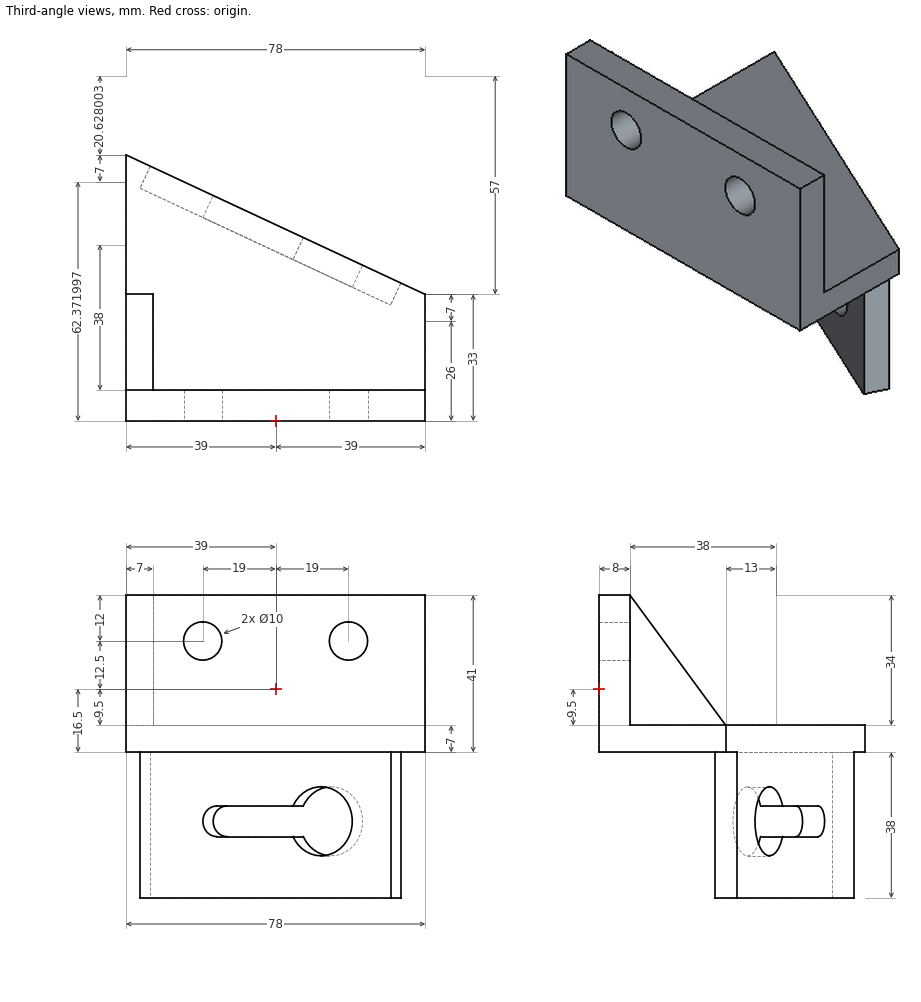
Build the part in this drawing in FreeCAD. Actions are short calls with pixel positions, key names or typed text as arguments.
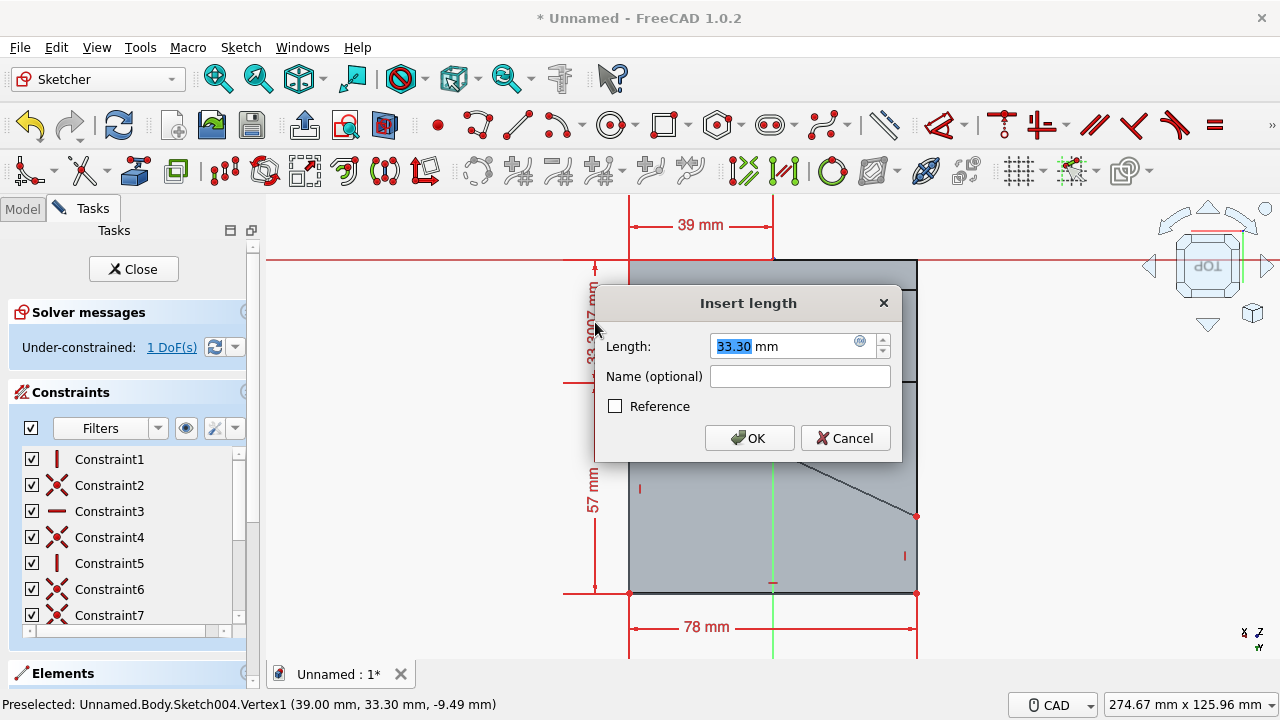
text(33)
key(Return)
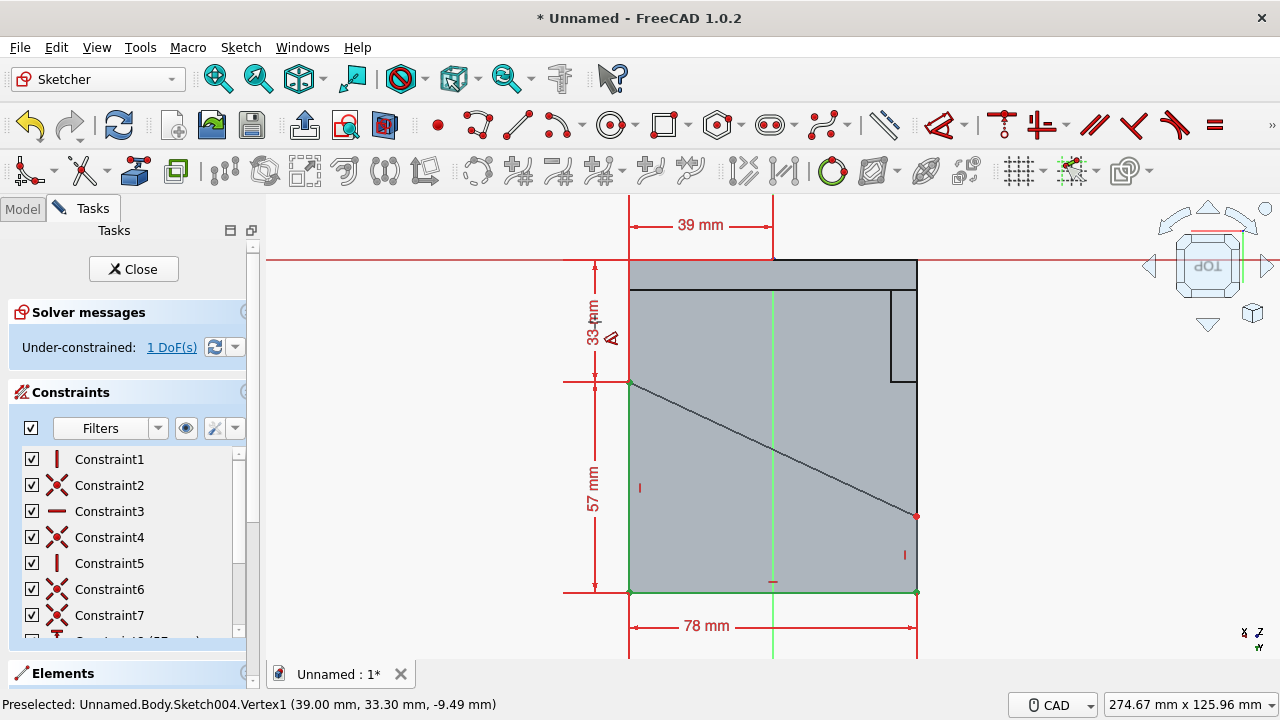
click(917, 570)
click(951, 555)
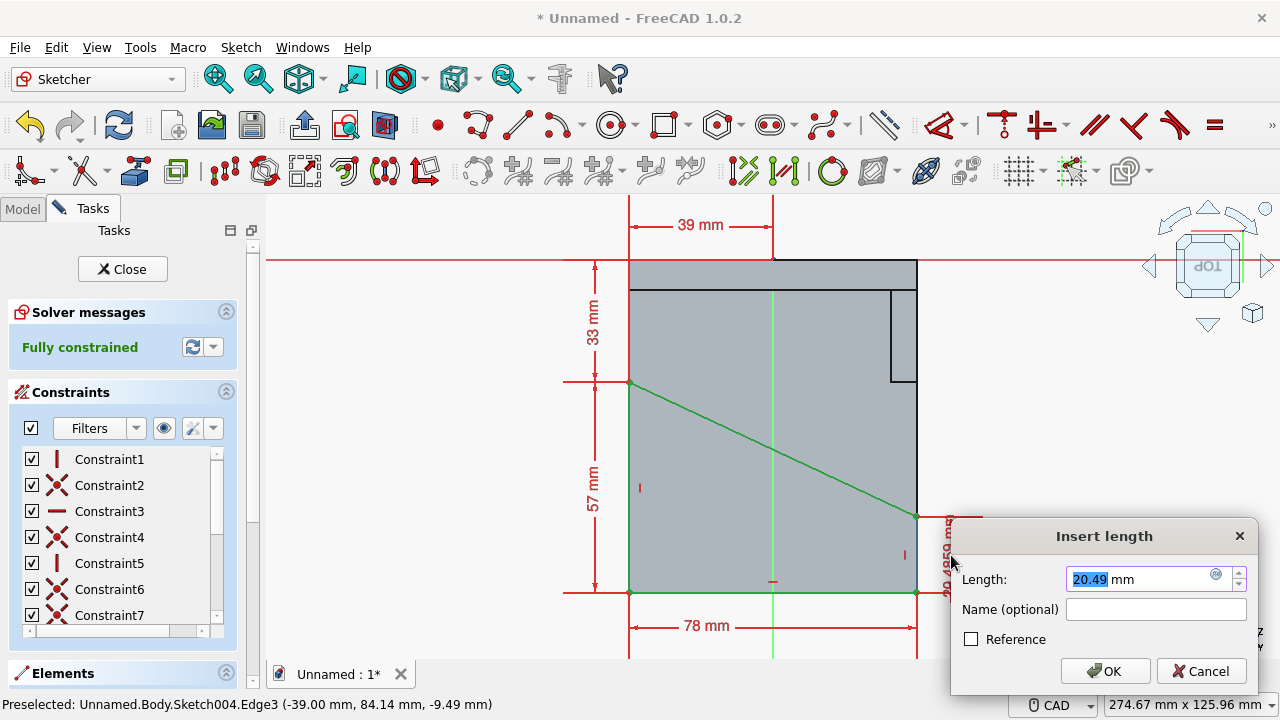
text(20.628003)
key(Return)
key(Escape)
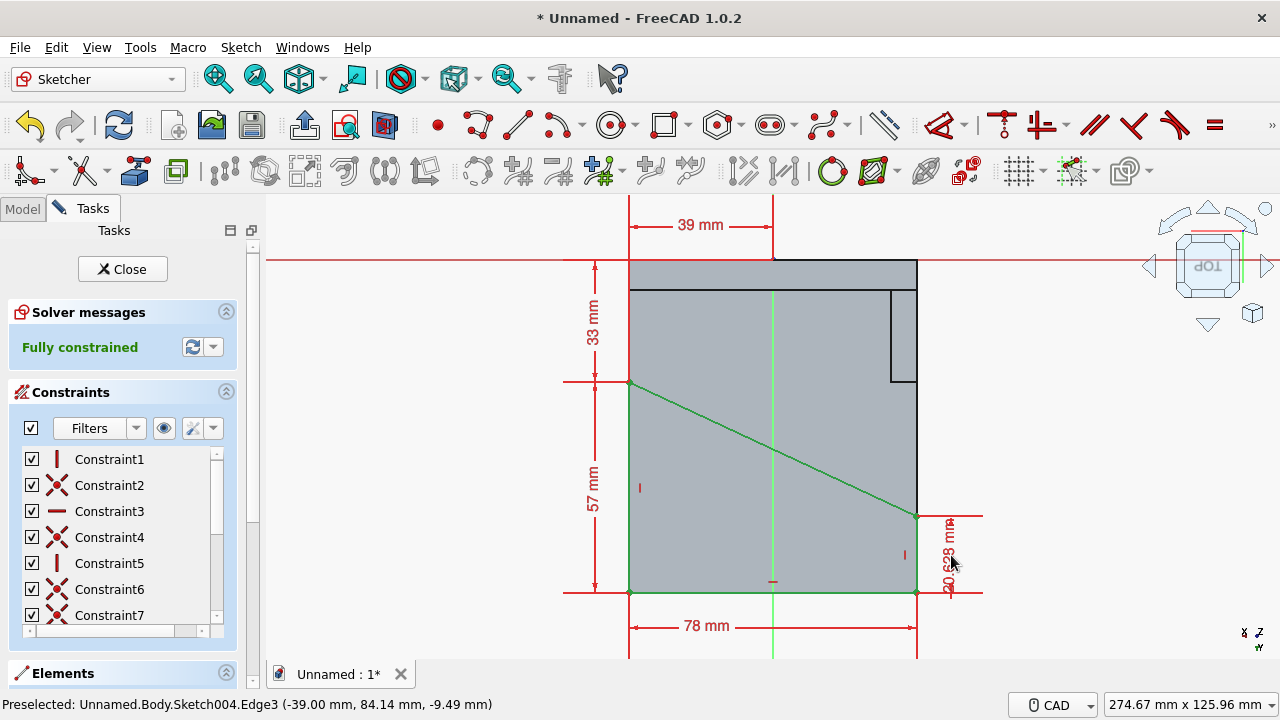
click(123, 269)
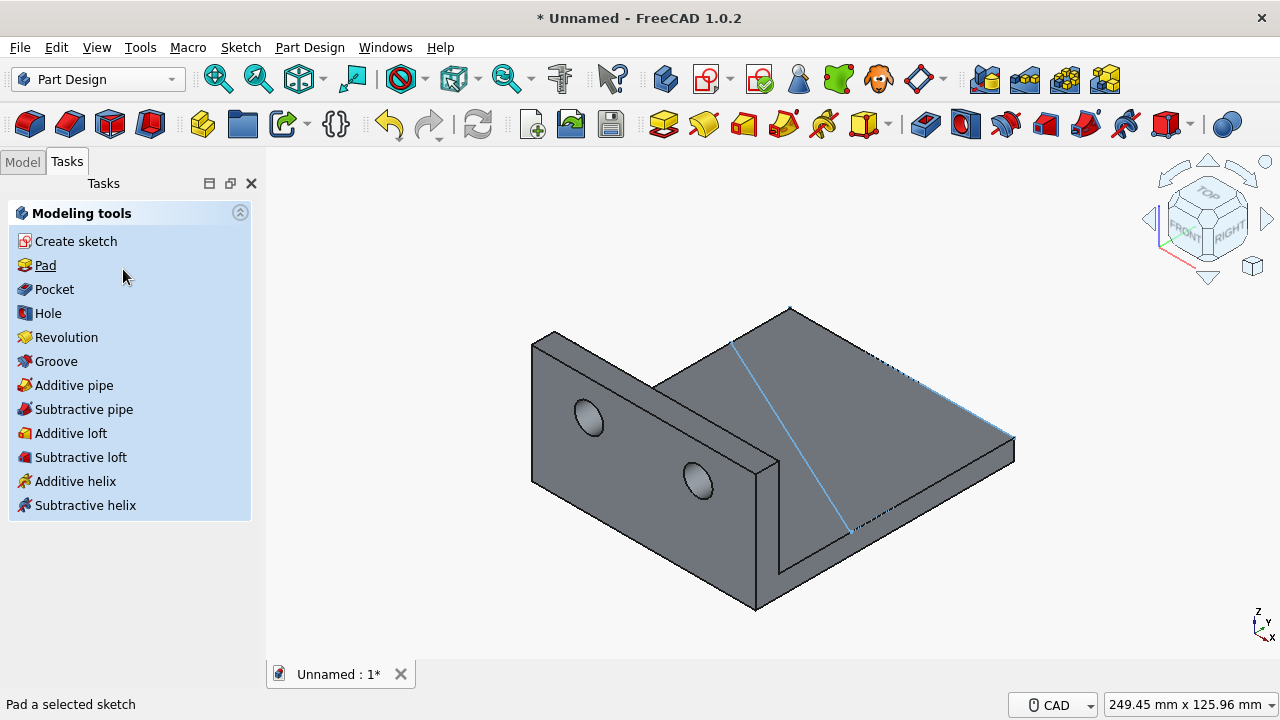
click(926, 124)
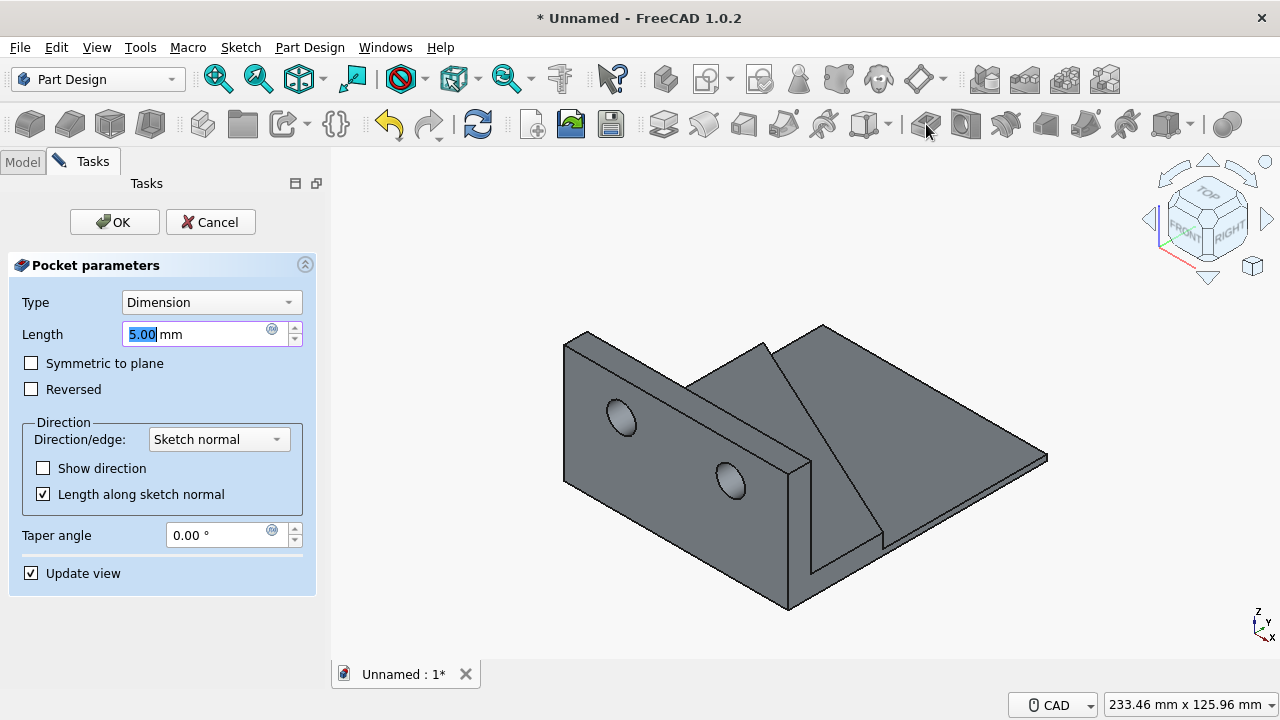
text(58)
key(Tab)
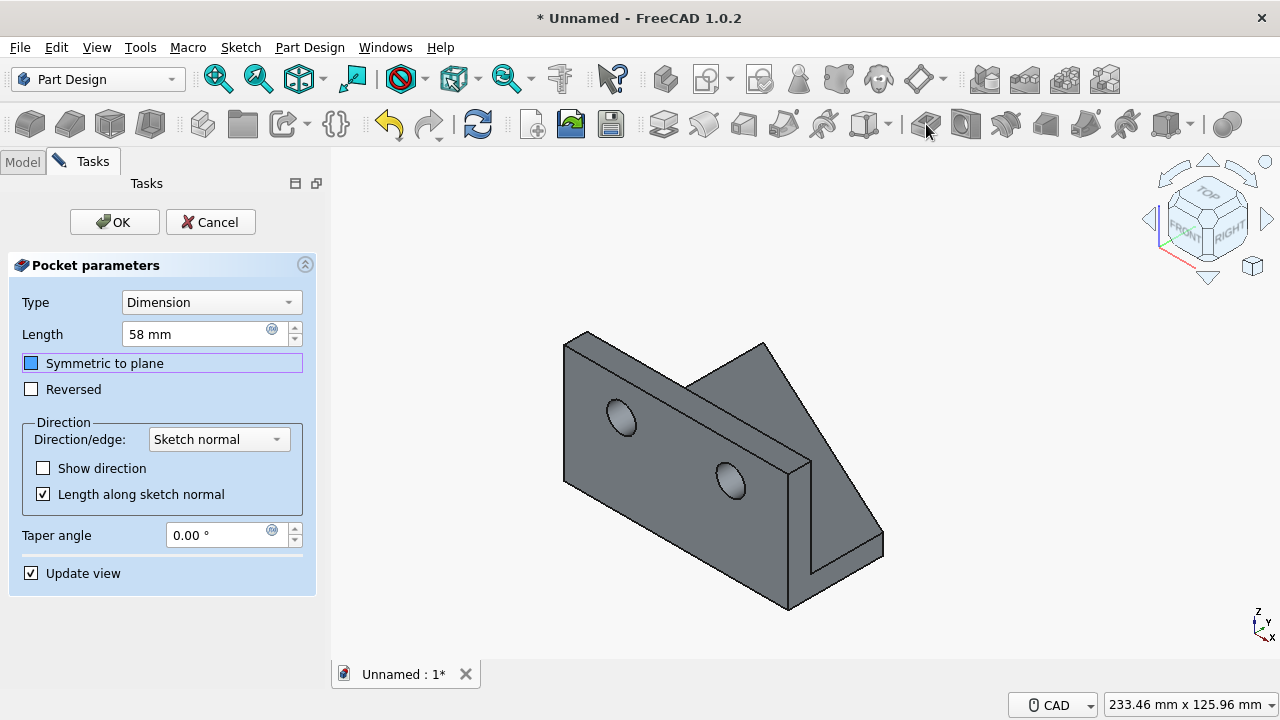
click(115, 222)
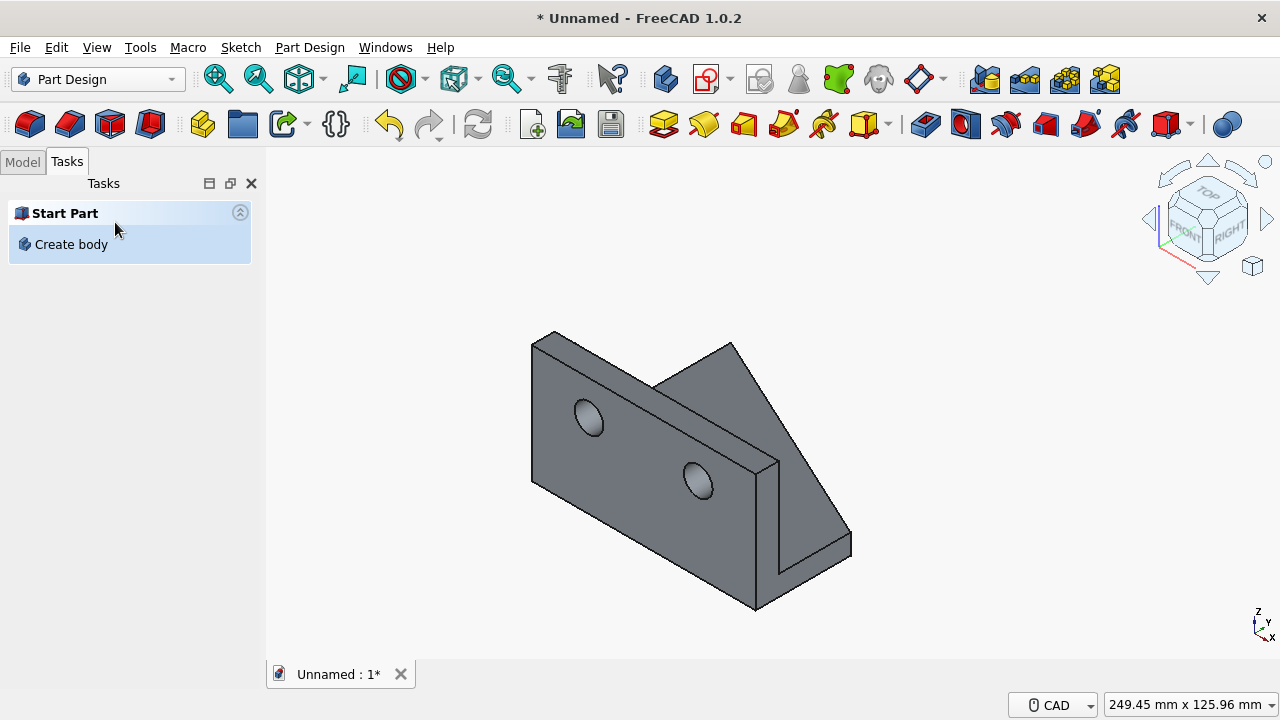
key(5)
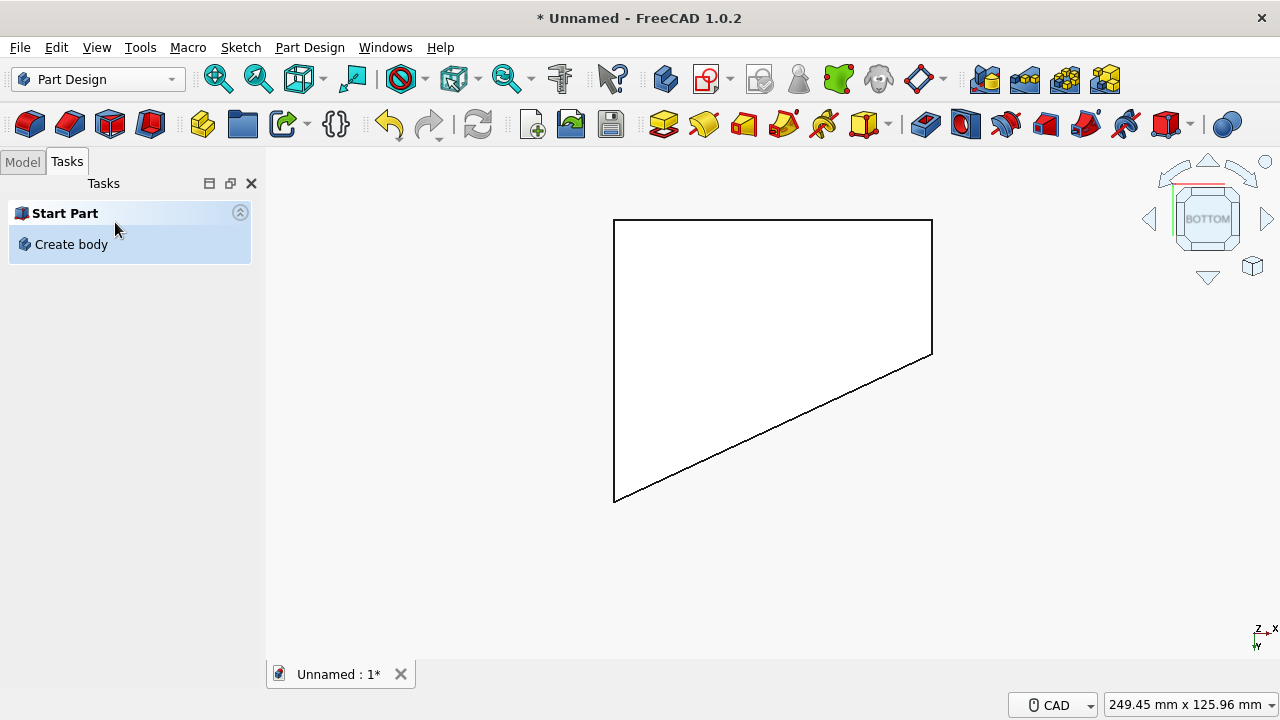
click(728, 320)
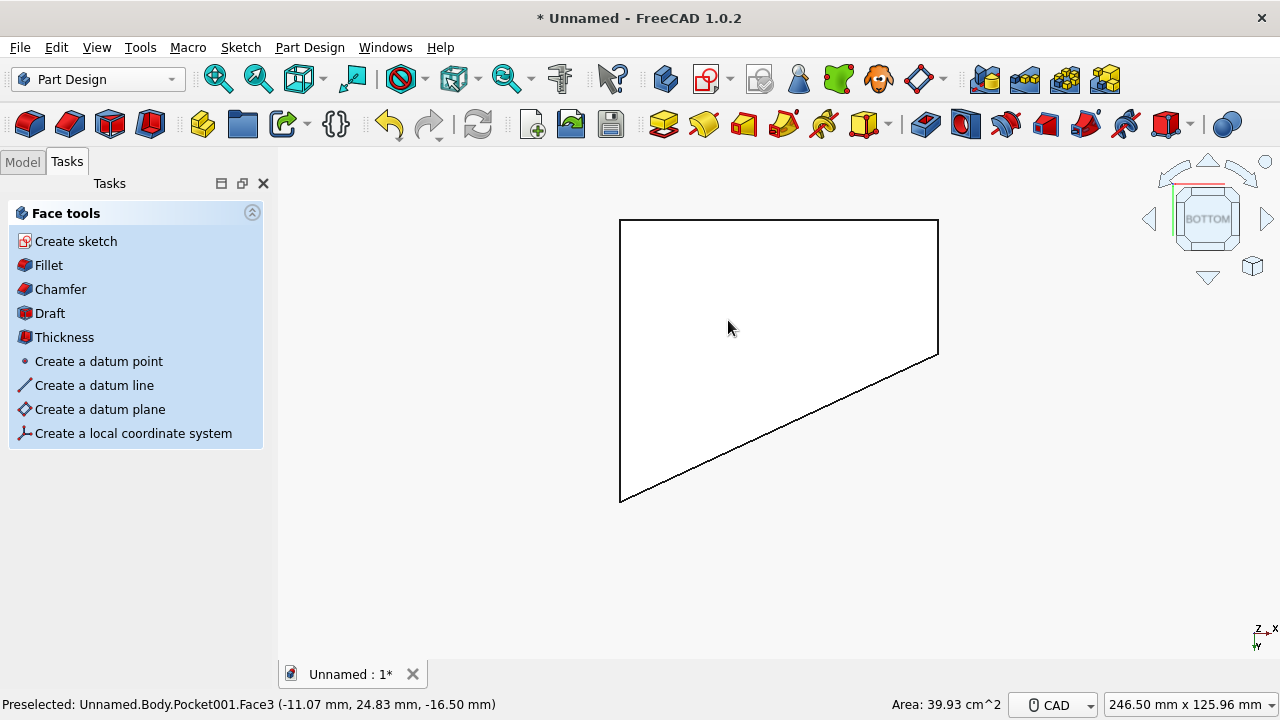
click(706, 80)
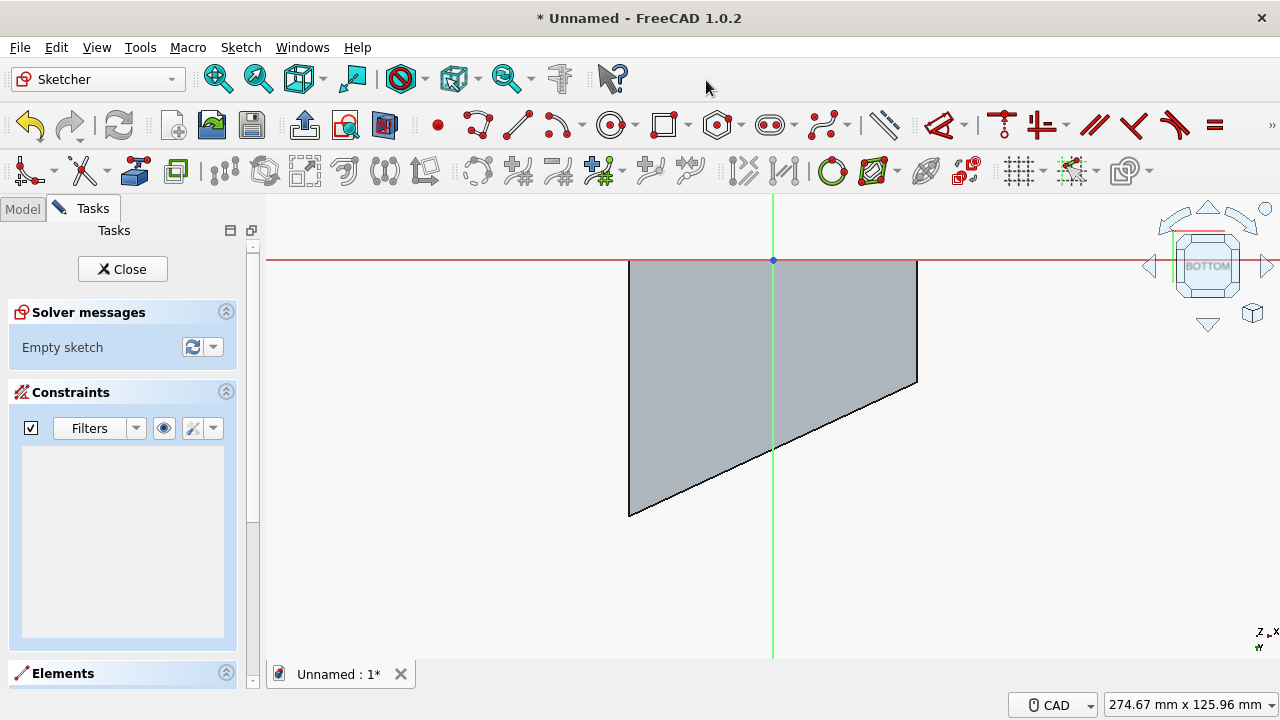
key(g)
key(m)